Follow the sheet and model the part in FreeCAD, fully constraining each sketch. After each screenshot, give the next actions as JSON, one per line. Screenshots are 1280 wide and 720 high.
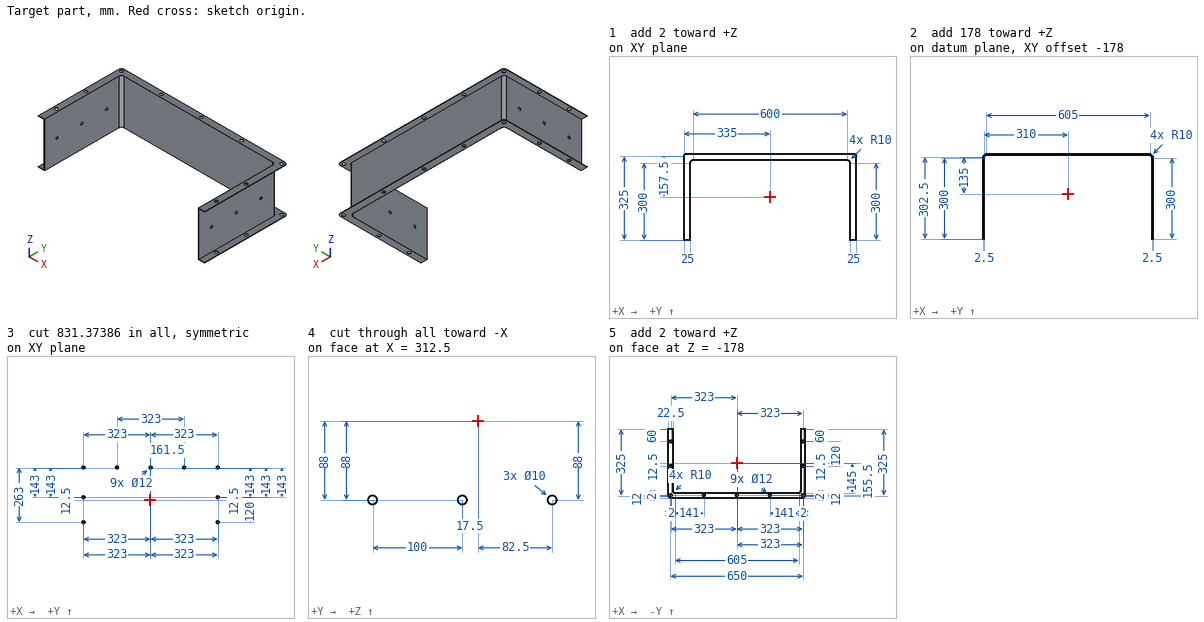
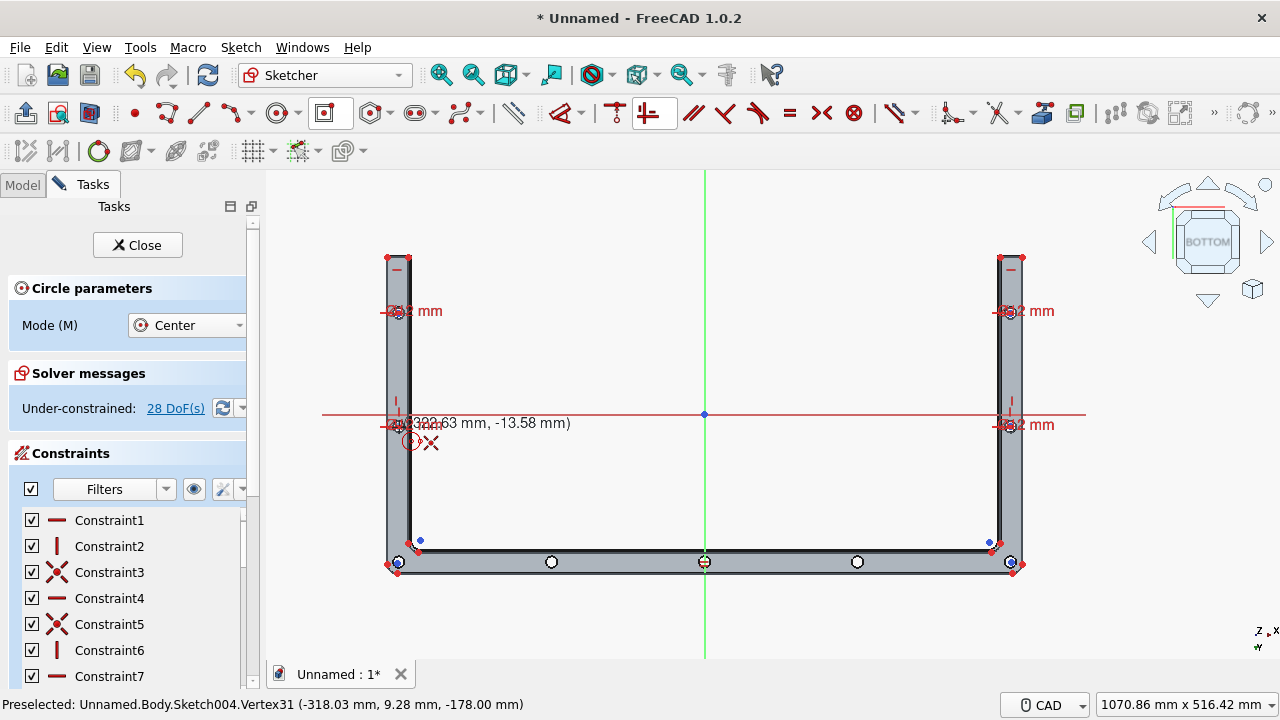
{"action": "scroll", "coordinate": [1010, 562], "scroll_direction": "up", "scroll_amount": 9}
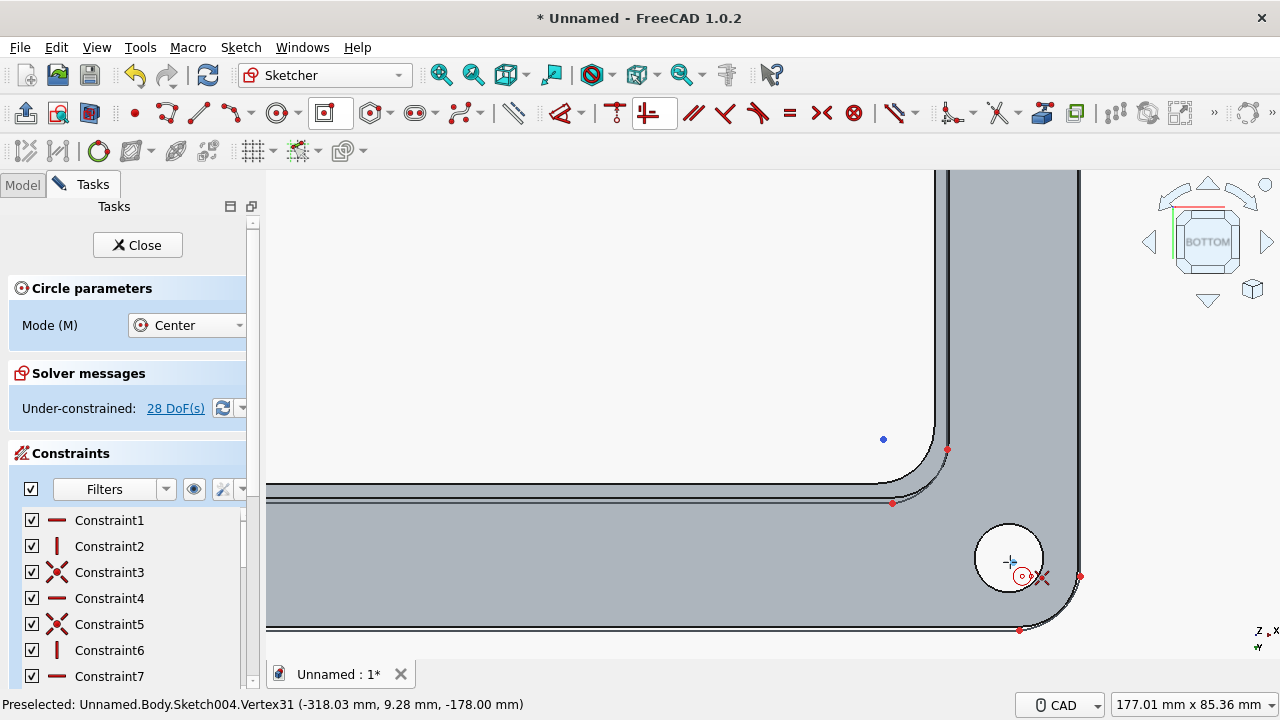
{"action": "left_click", "coordinate": [1009, 558]}
{"action": "mouse_move", "coordinate": [1033, 534]}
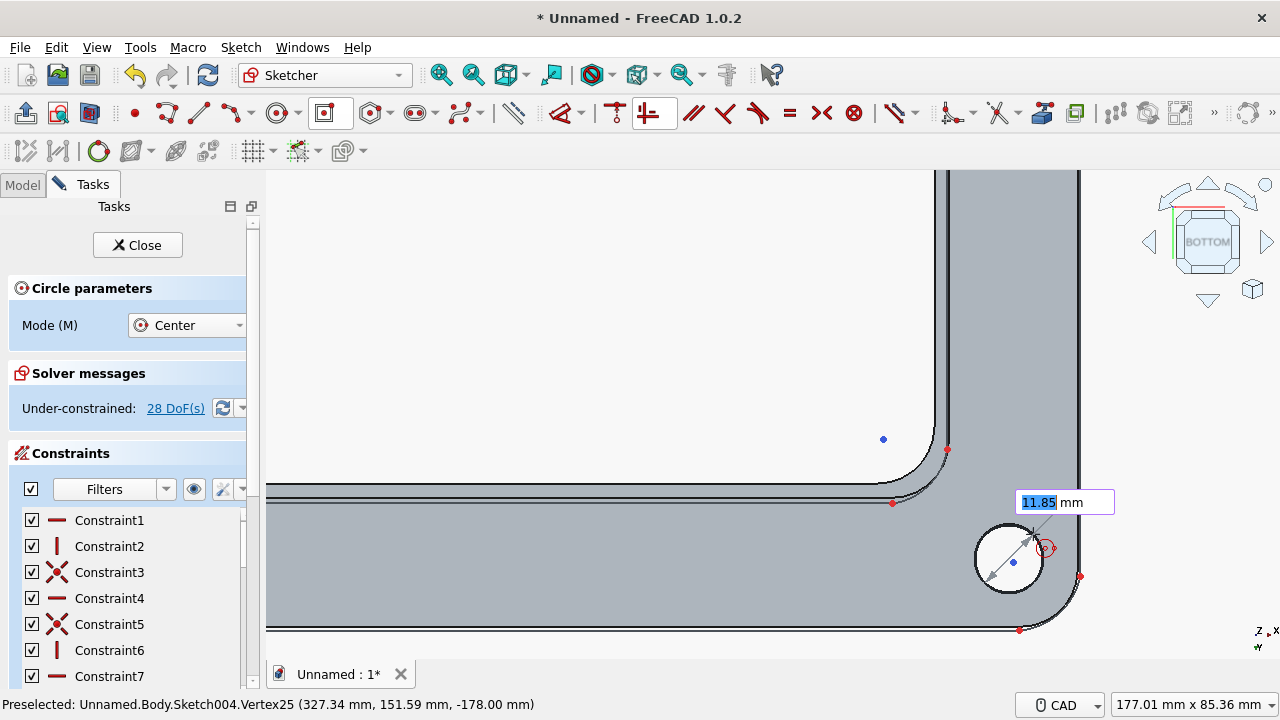
{"action": "type", "text": "12"}
{"action": "key", "text": "Return"}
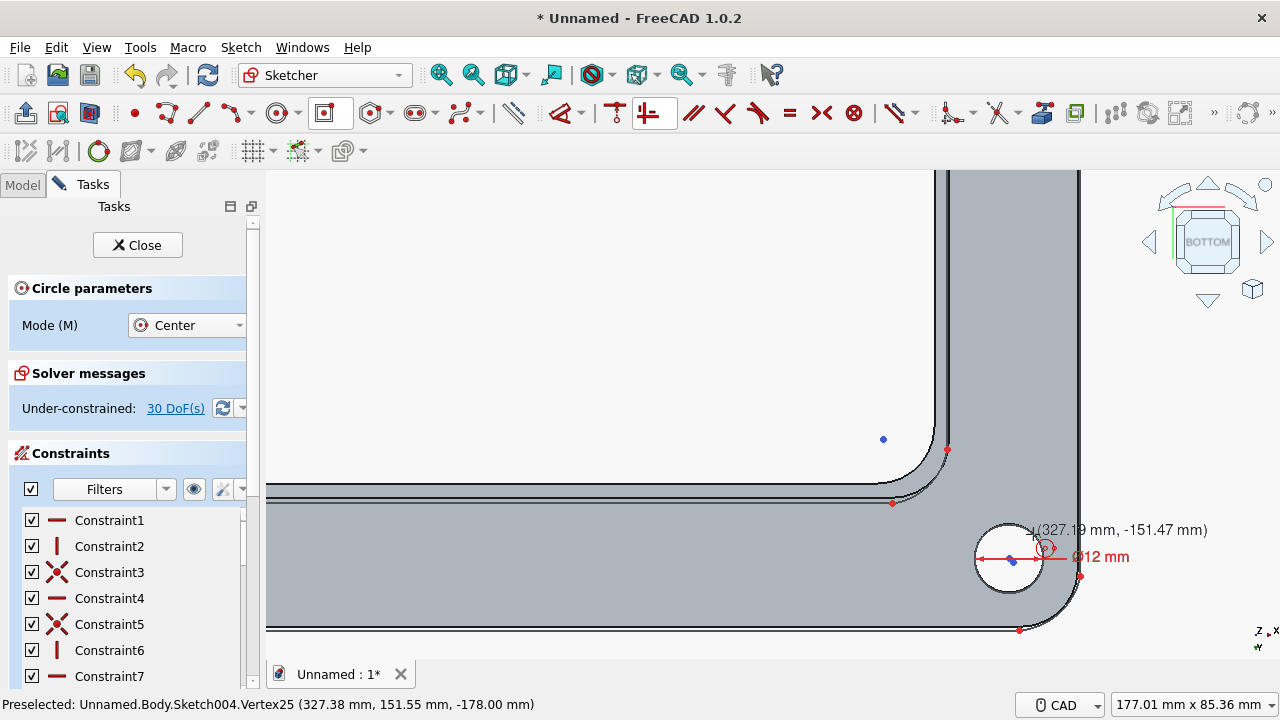
{"action": "scroll", "coordinate": [1011, 562], "scroll_direction": "down", "scroll_amount": 9}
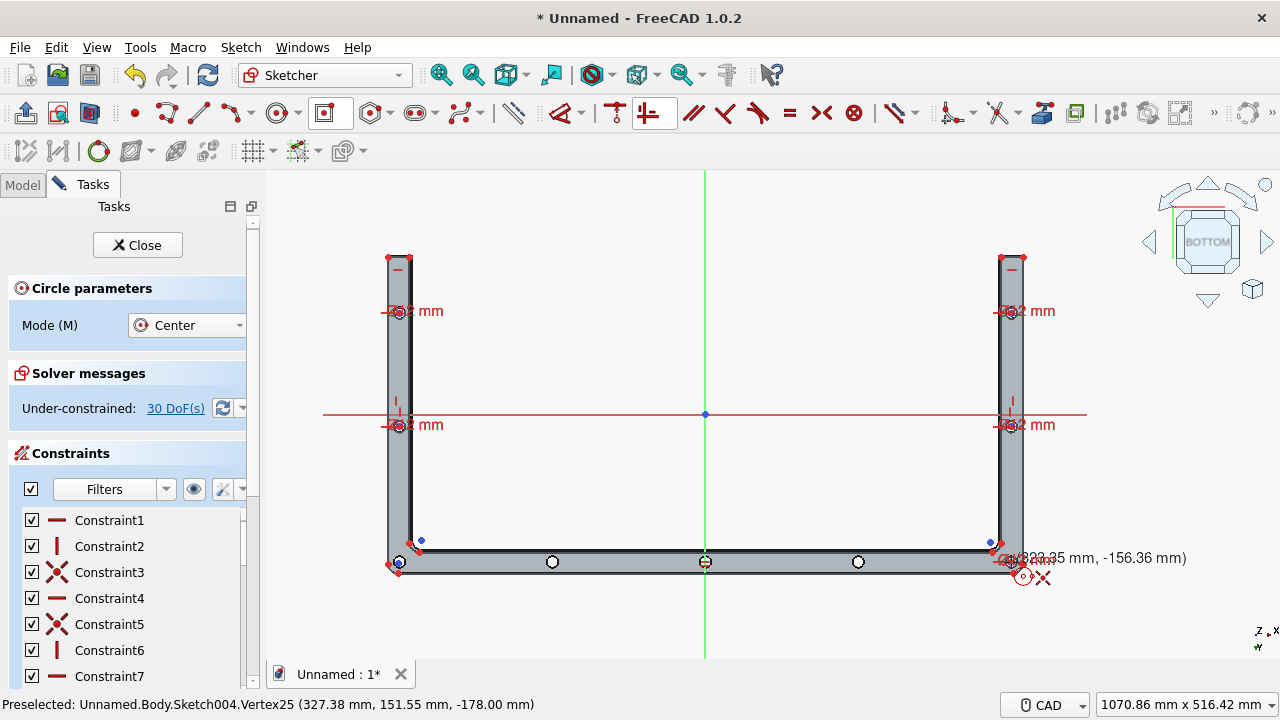
{"action": "scroll", "coordinate": [858, 562], "scroll_direction": "up", "scroll_amount": 7}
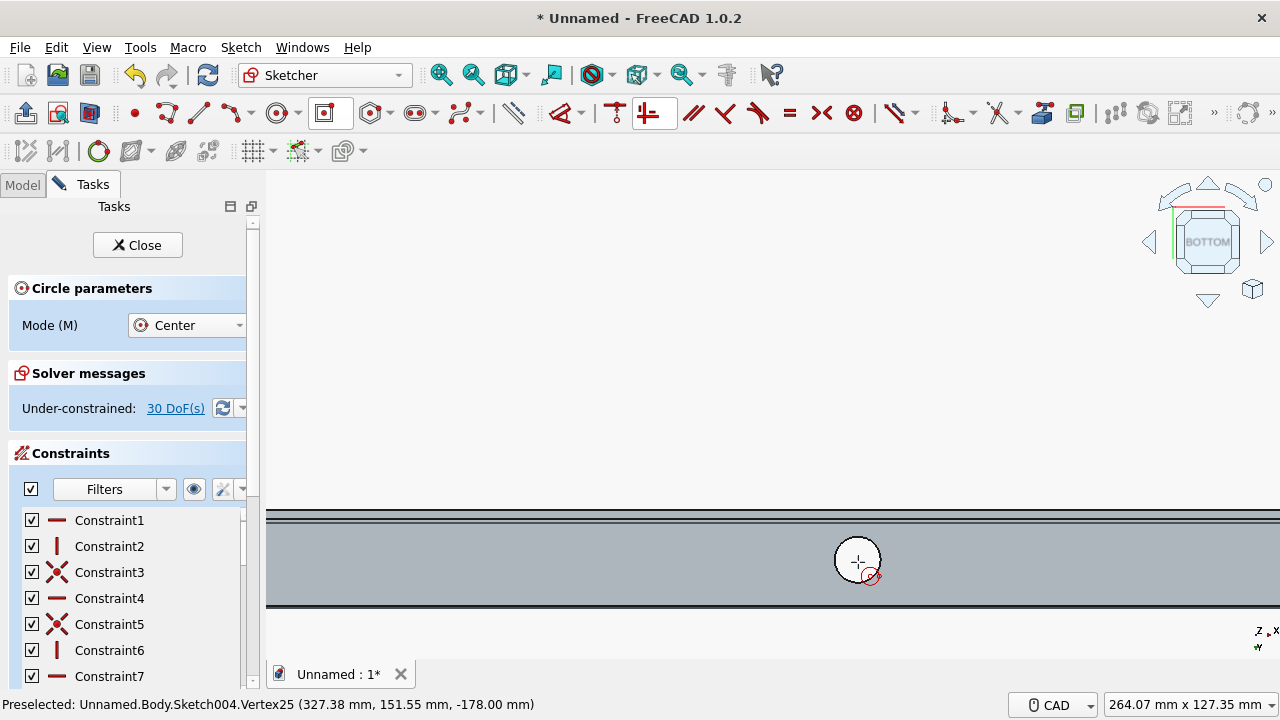
{"action": "left_click", "coordinate": [858, 560]}
{"action": "mouse_move", "coordinate": [874, 543]}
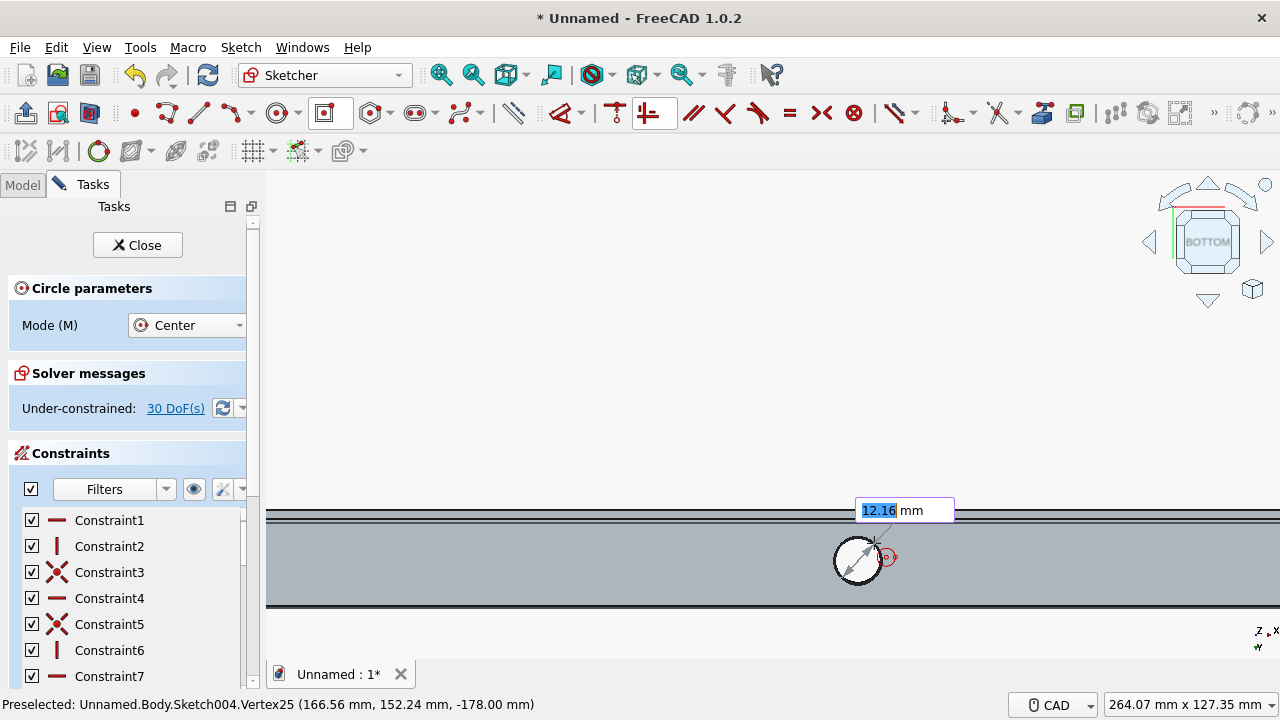
{"action": "type", "text": "12"}
{"action": "key", "text": "Return"}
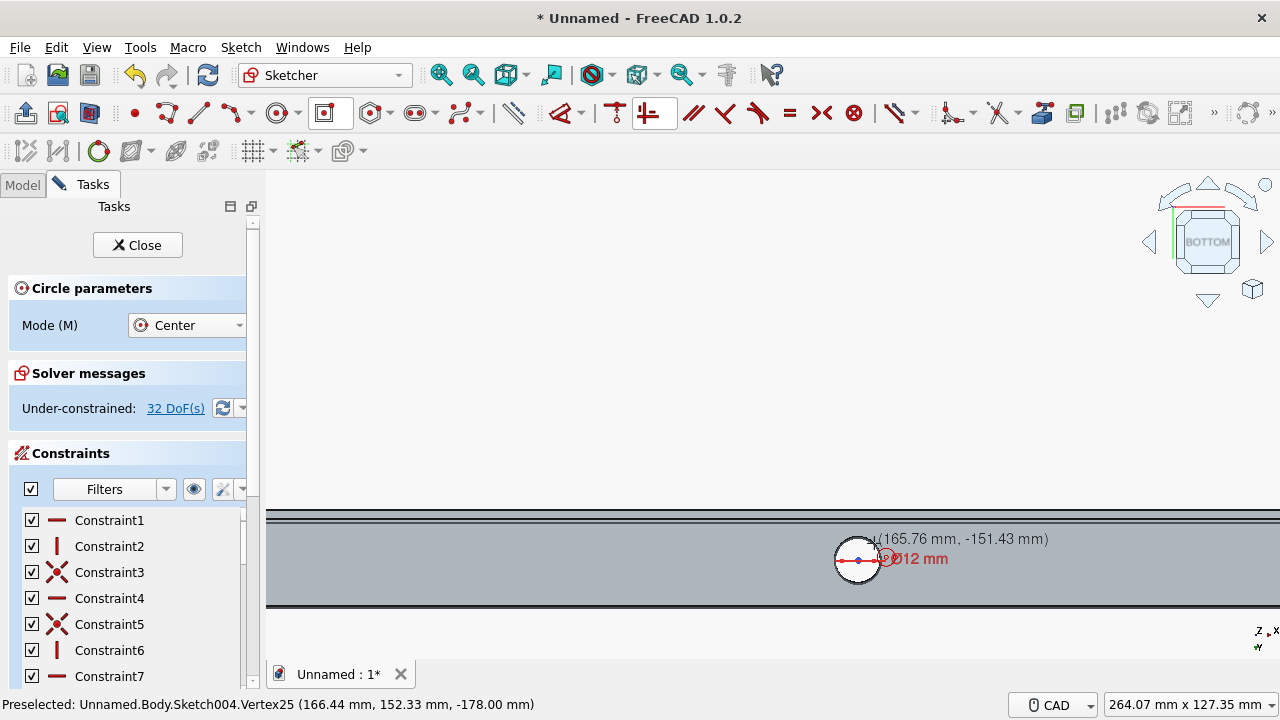
{"action": "scroll", "coordinate": [857, 562], "scroll_direction": "down", "scroll_amount": 7}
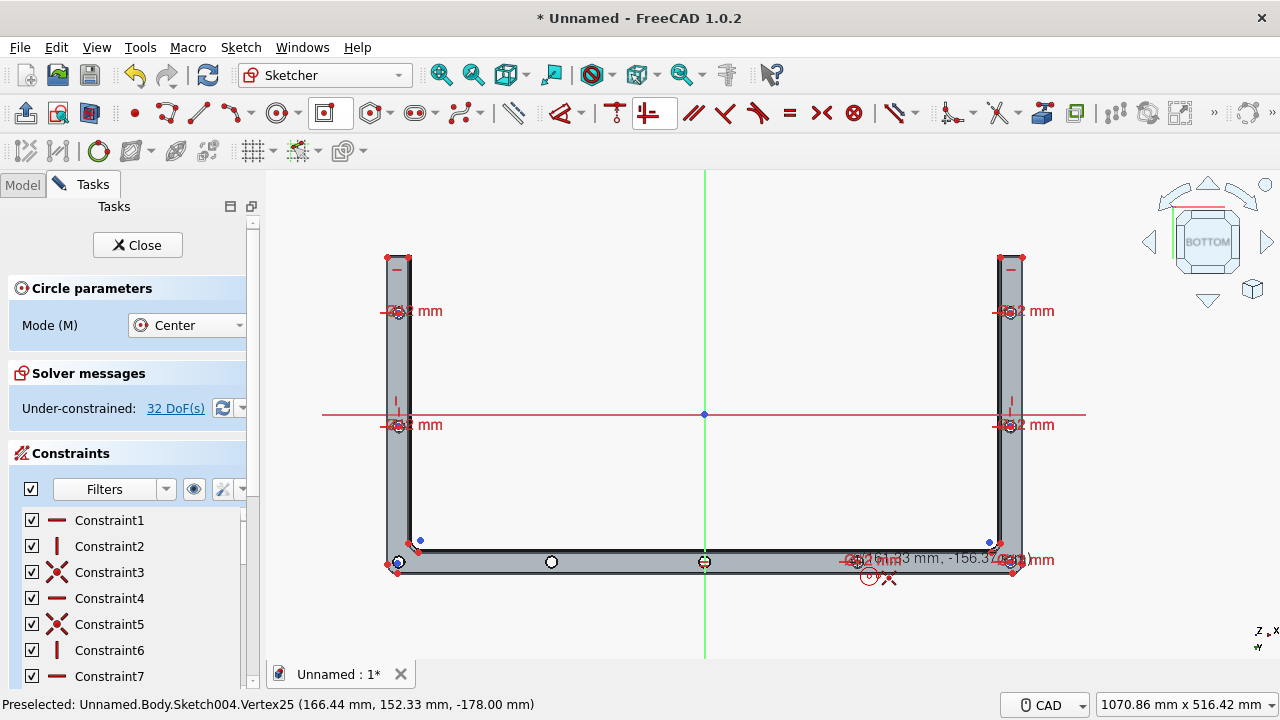
{"action": "scroll", "coordinate": [705, 562], "scroll_direction": "up", "scroll_amount": 7}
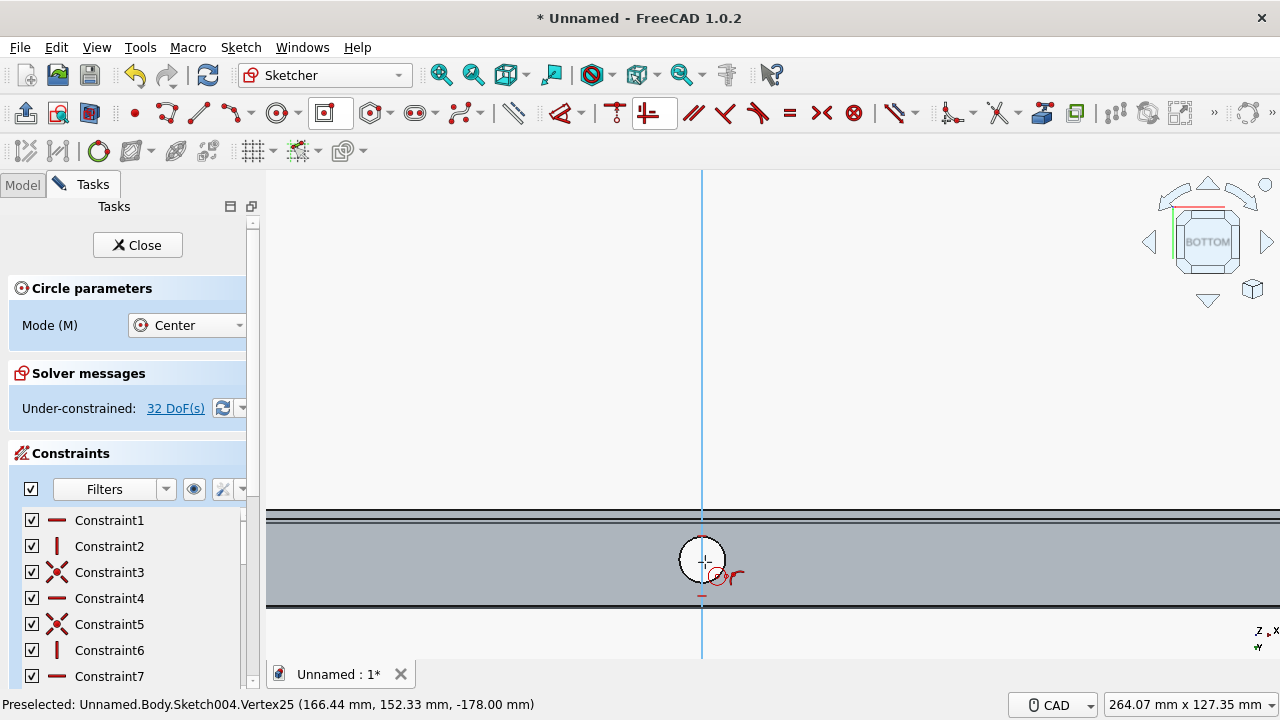
{"action": "left_click", "coordinate": [702, 560]}
{"action": "mouse_move", "coordinate": [719, 543]}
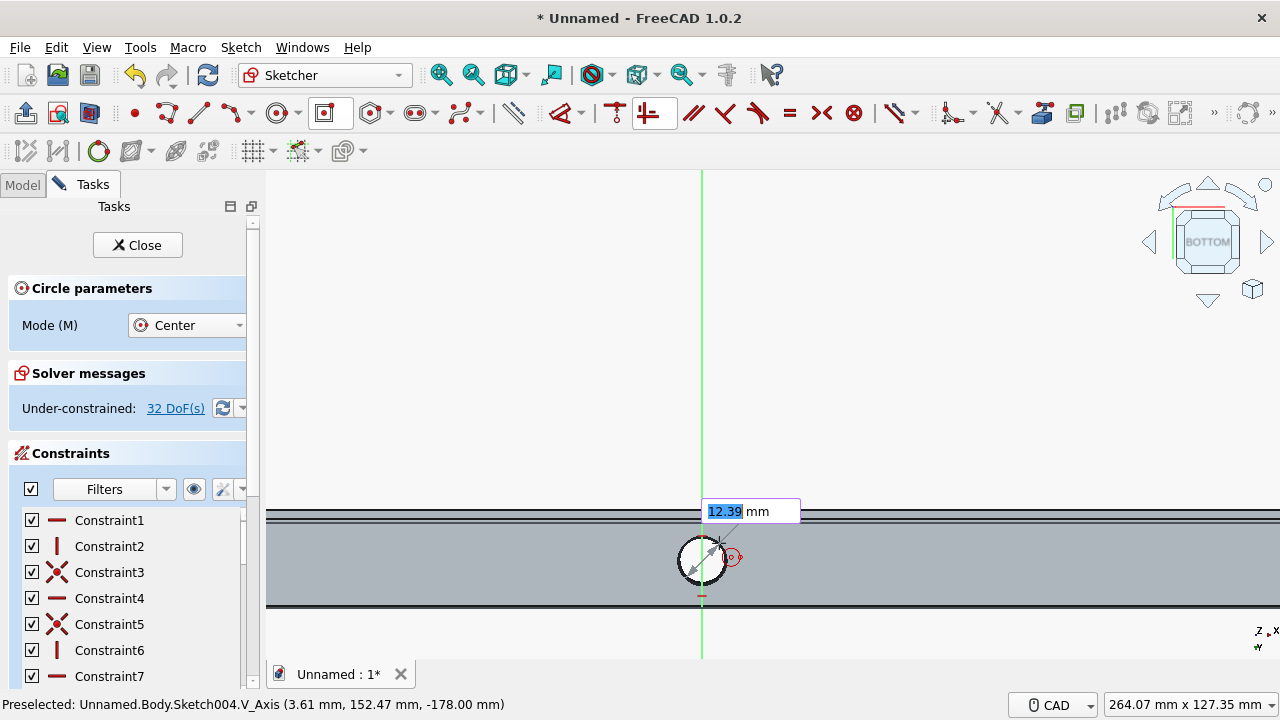
{"action": "type", "text": "12"}
{"action": "key", "text": "Return"}